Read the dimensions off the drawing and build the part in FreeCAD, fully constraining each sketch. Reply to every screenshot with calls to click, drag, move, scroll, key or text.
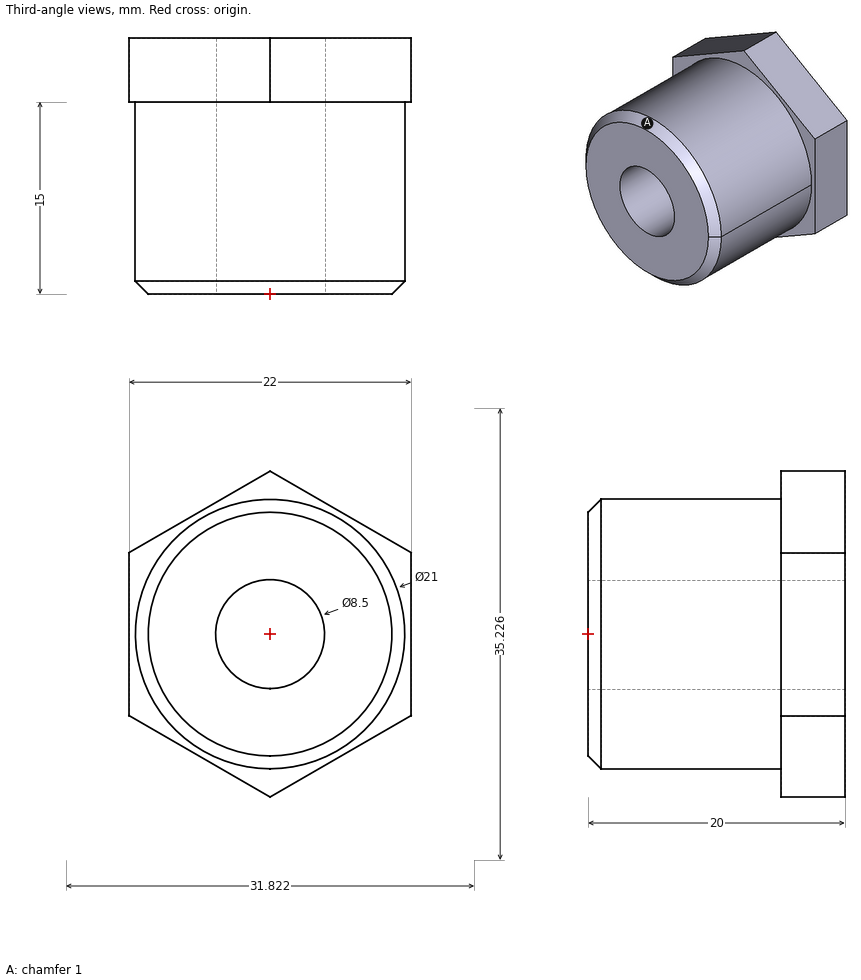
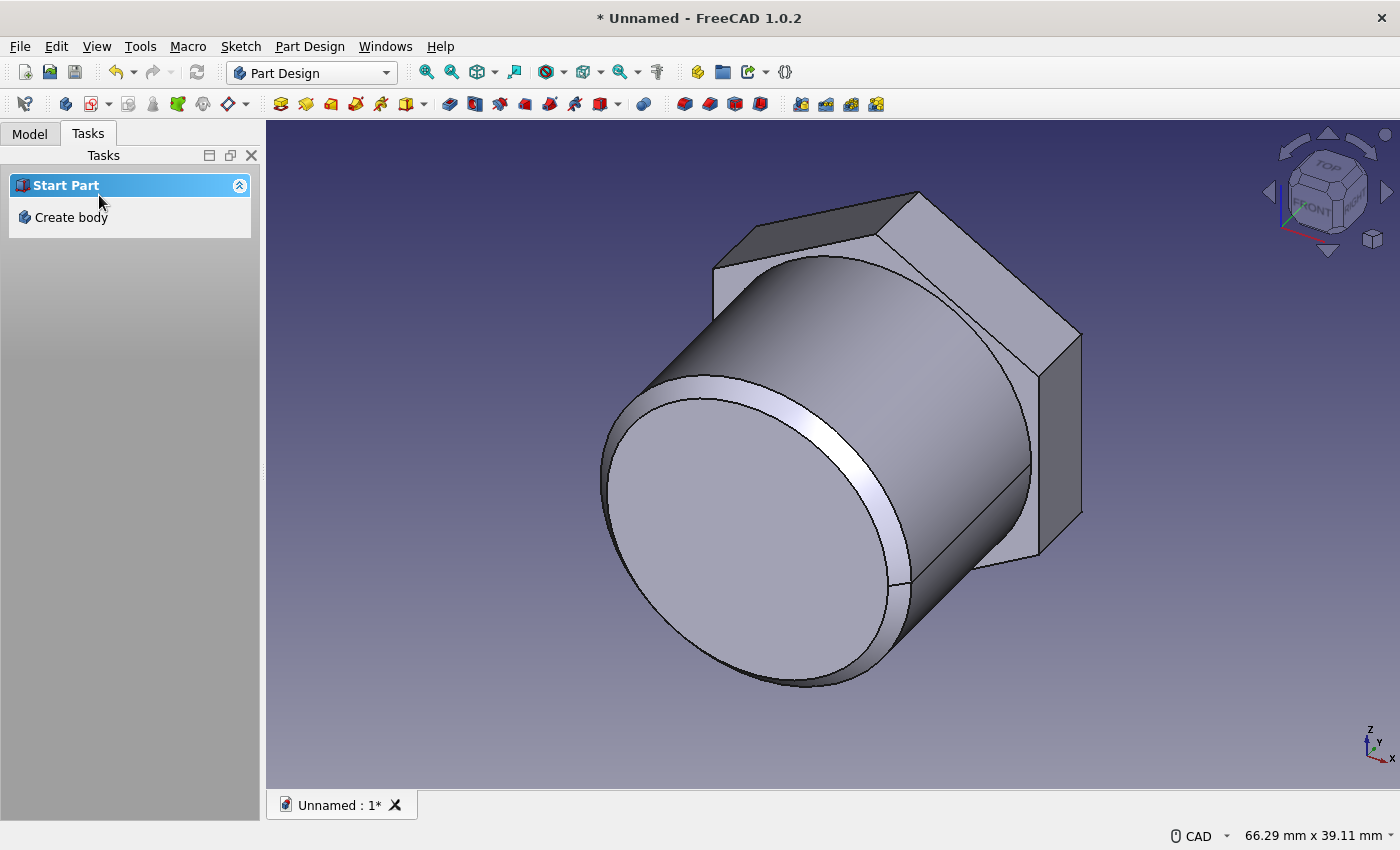
key(4)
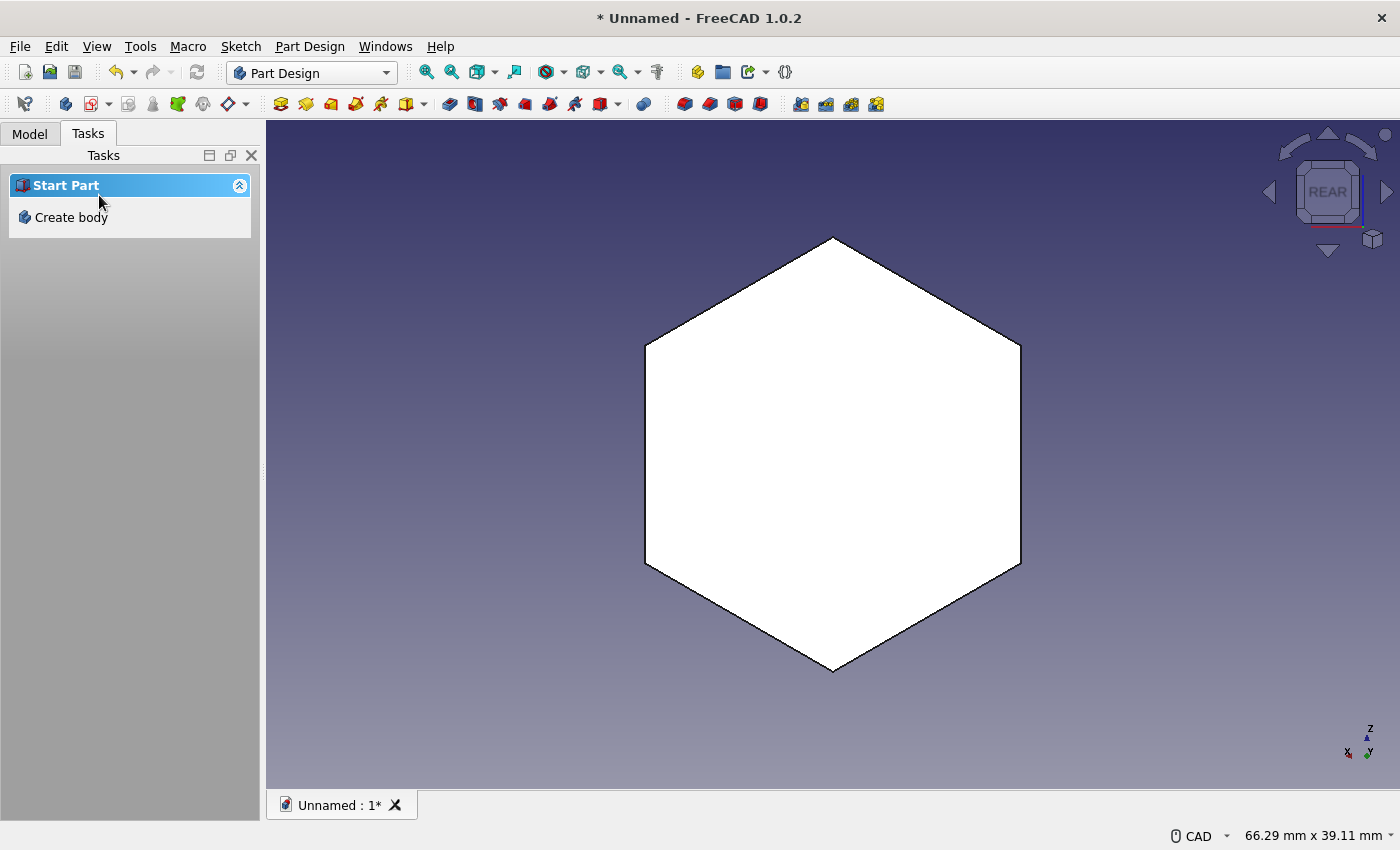
click(833, 454)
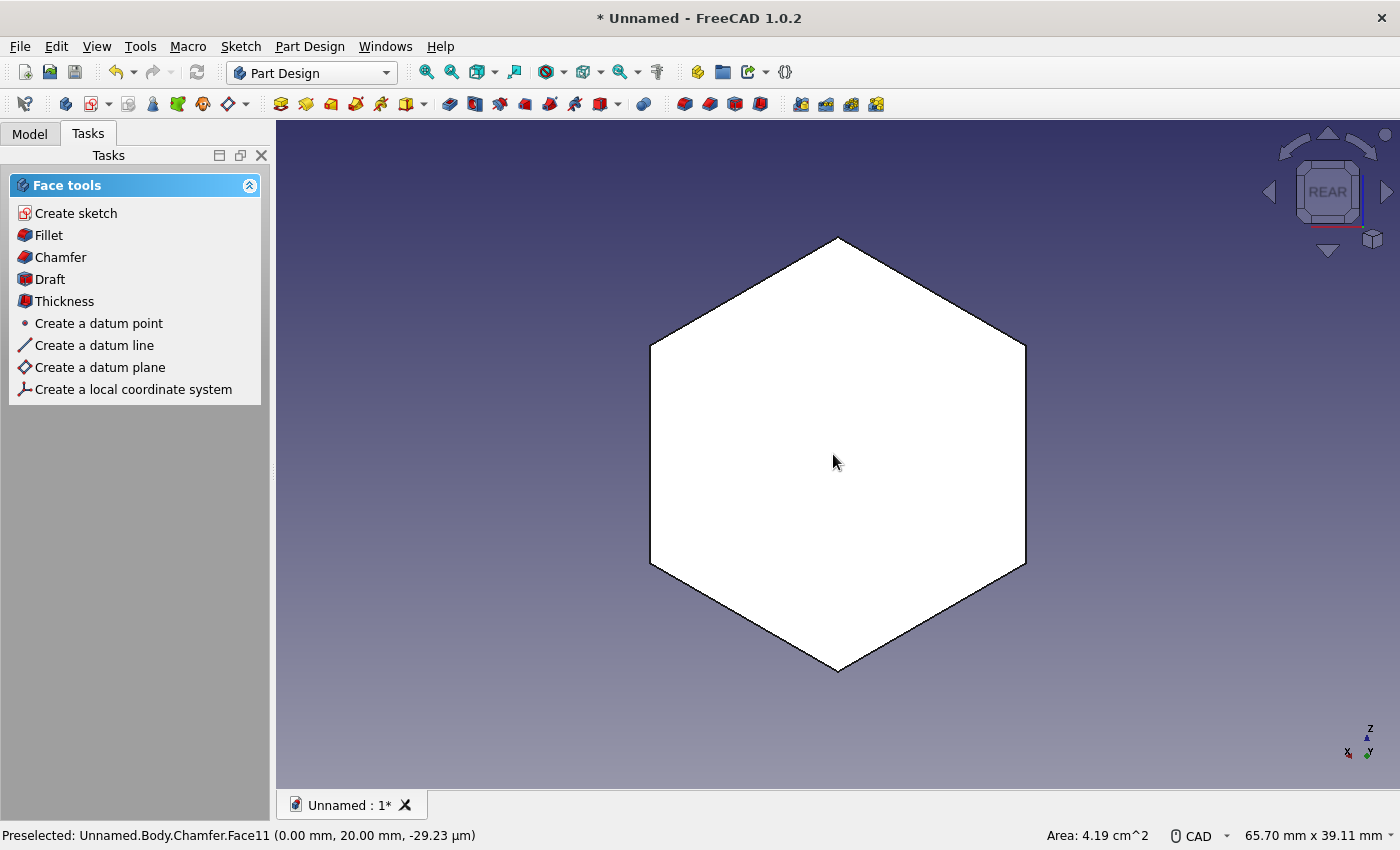
click(90, 104)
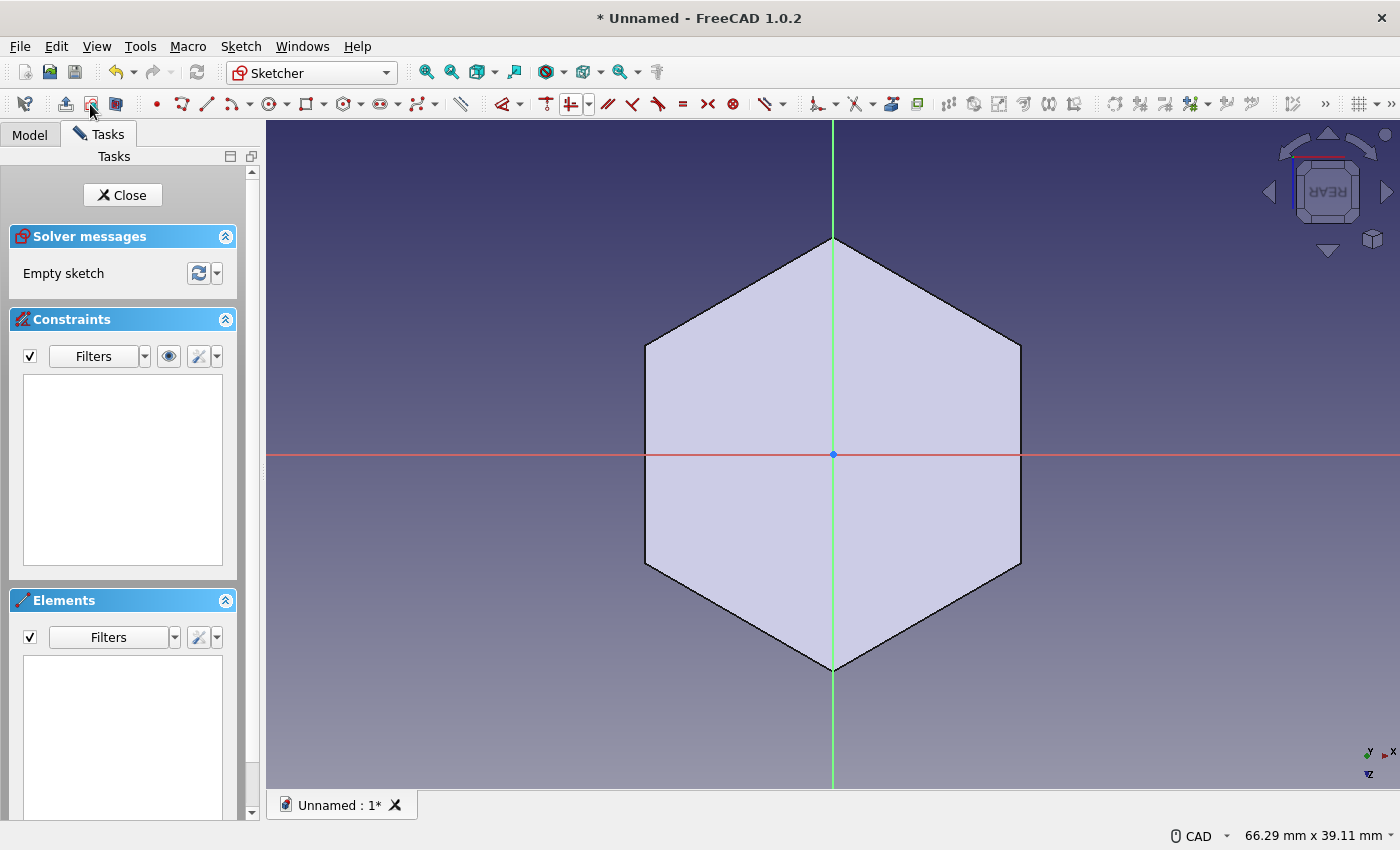
scroll(873, 455, up, 5)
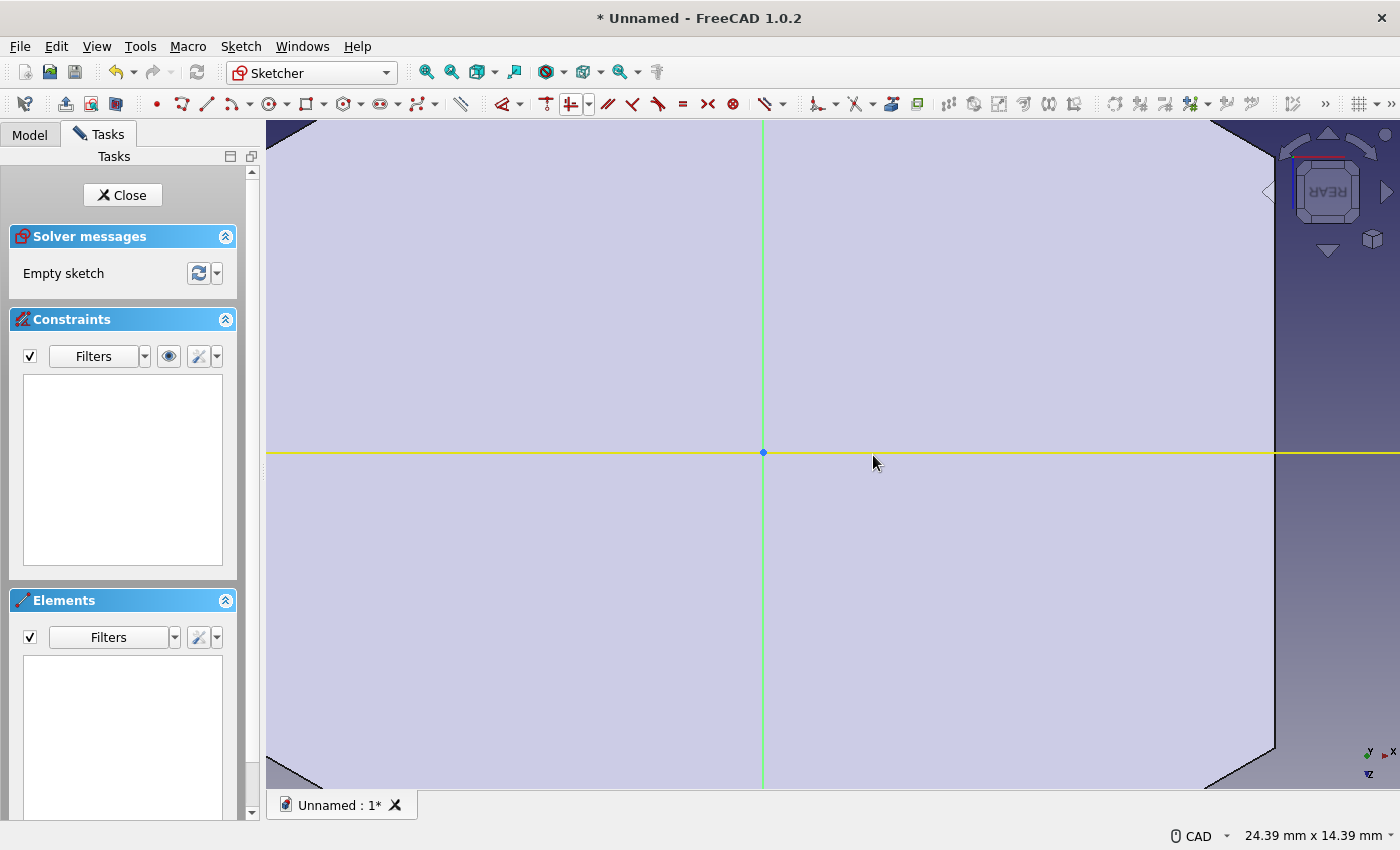
key(g)
key(c)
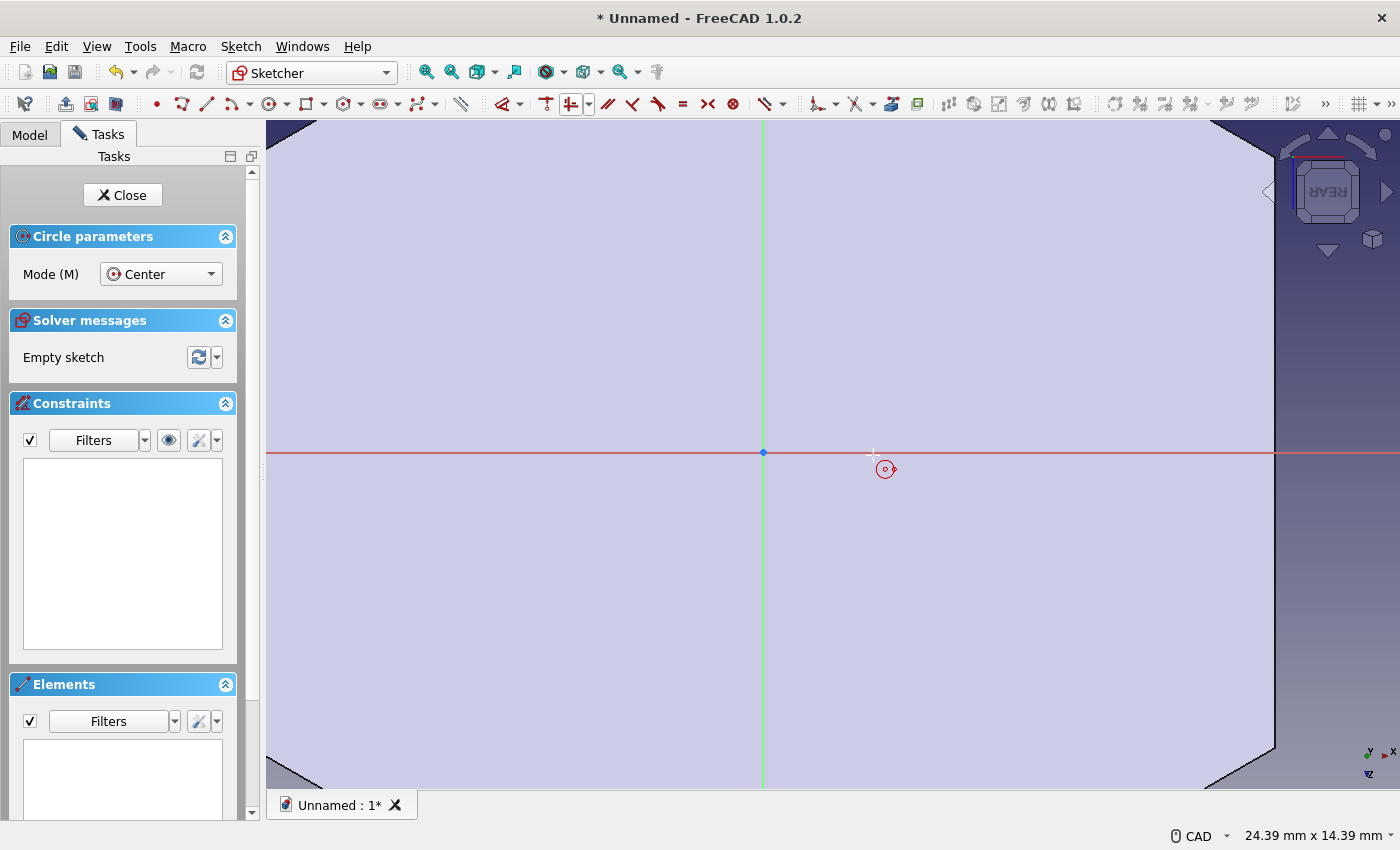
click(763, 453)
move(903, 313)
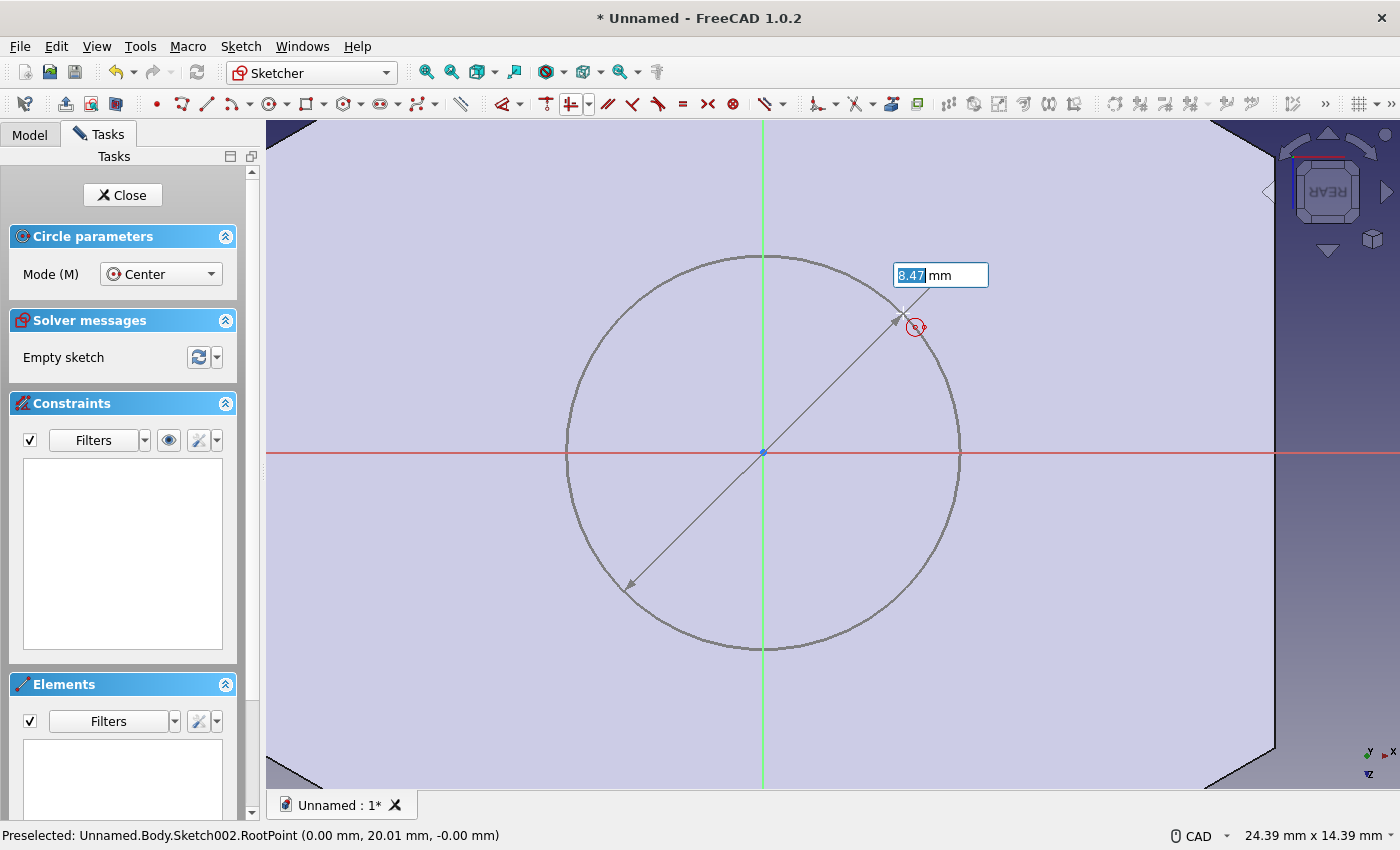
text(8.5)
key(Return)
key(Escape)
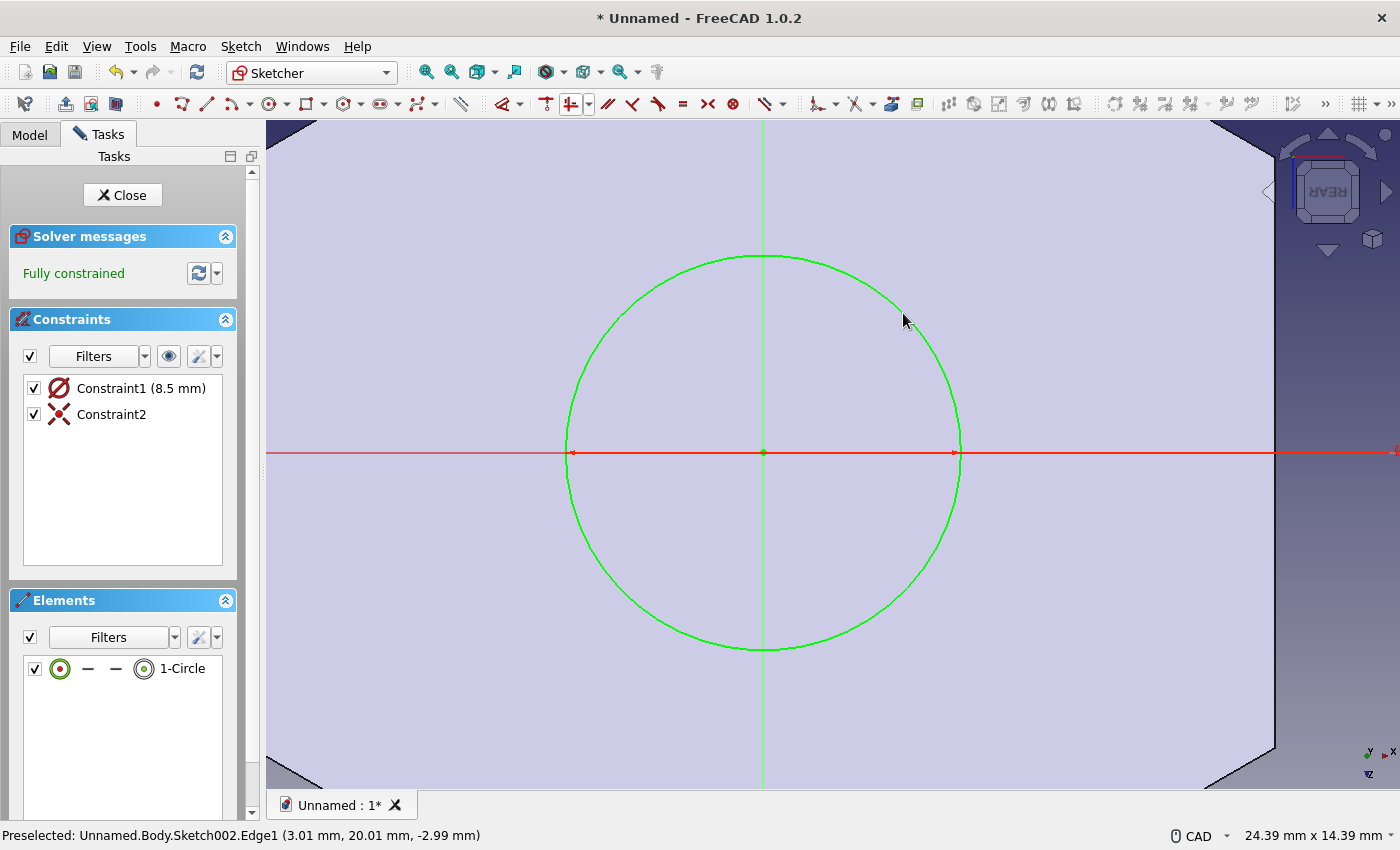
click(123, 195)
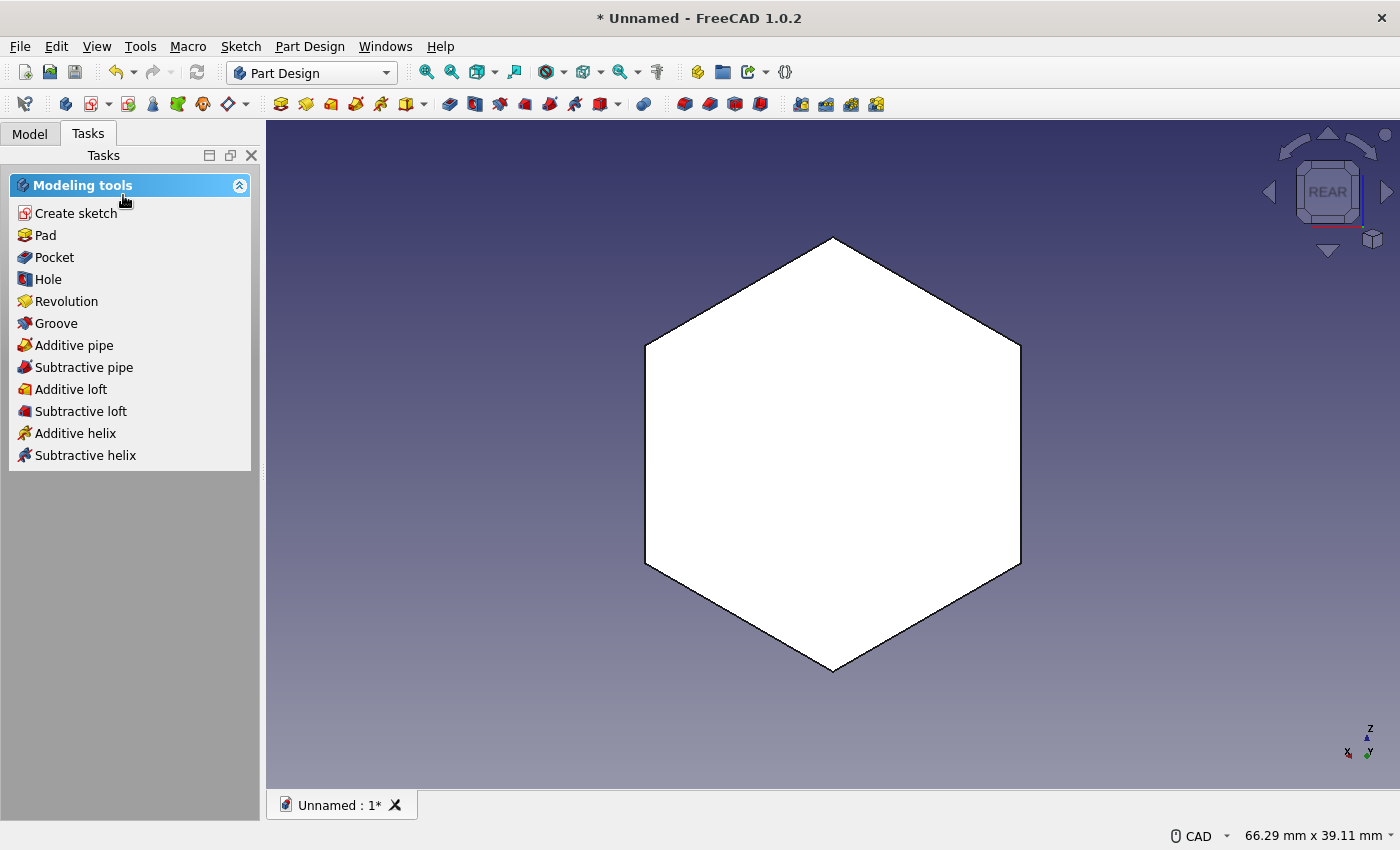
click(450, 104)